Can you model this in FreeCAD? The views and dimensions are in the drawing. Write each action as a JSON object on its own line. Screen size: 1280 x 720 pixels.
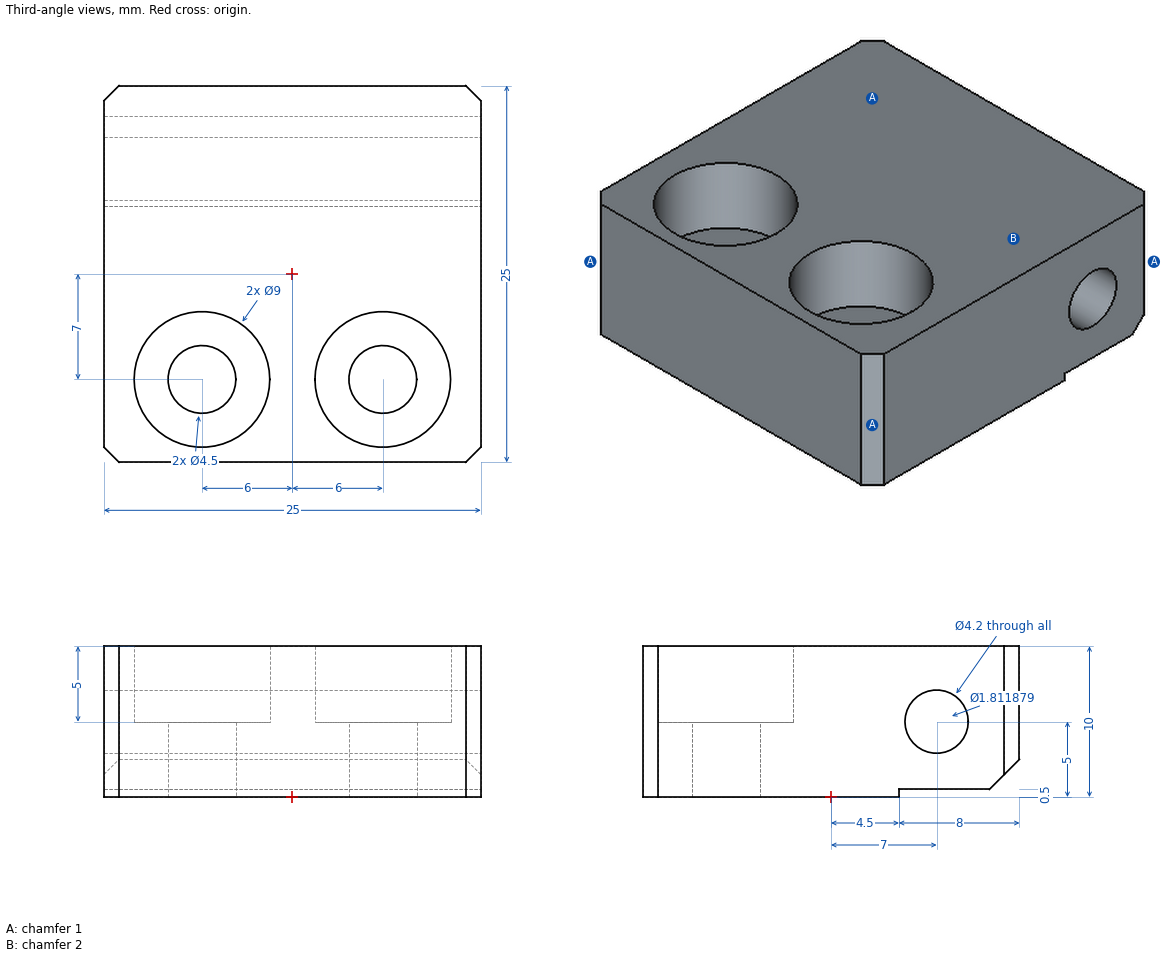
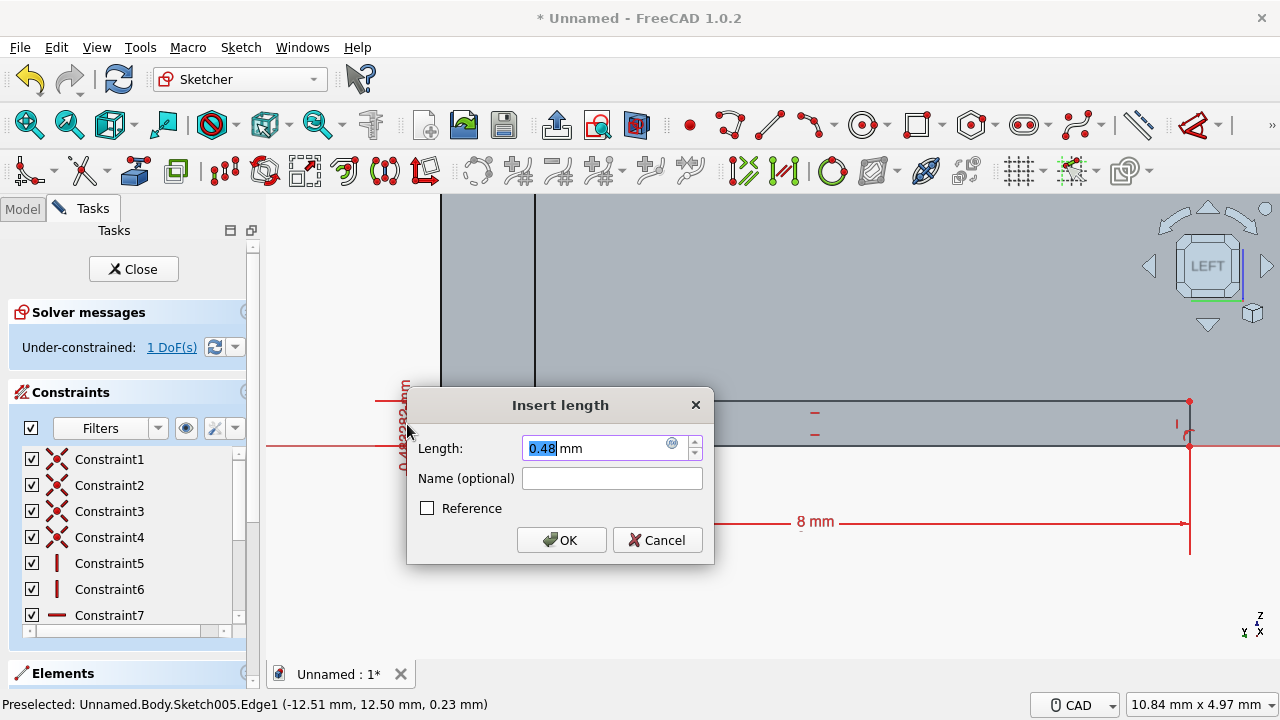
{"action": "type", "text": "0.5"}
{"action": "key", "text": "Return"}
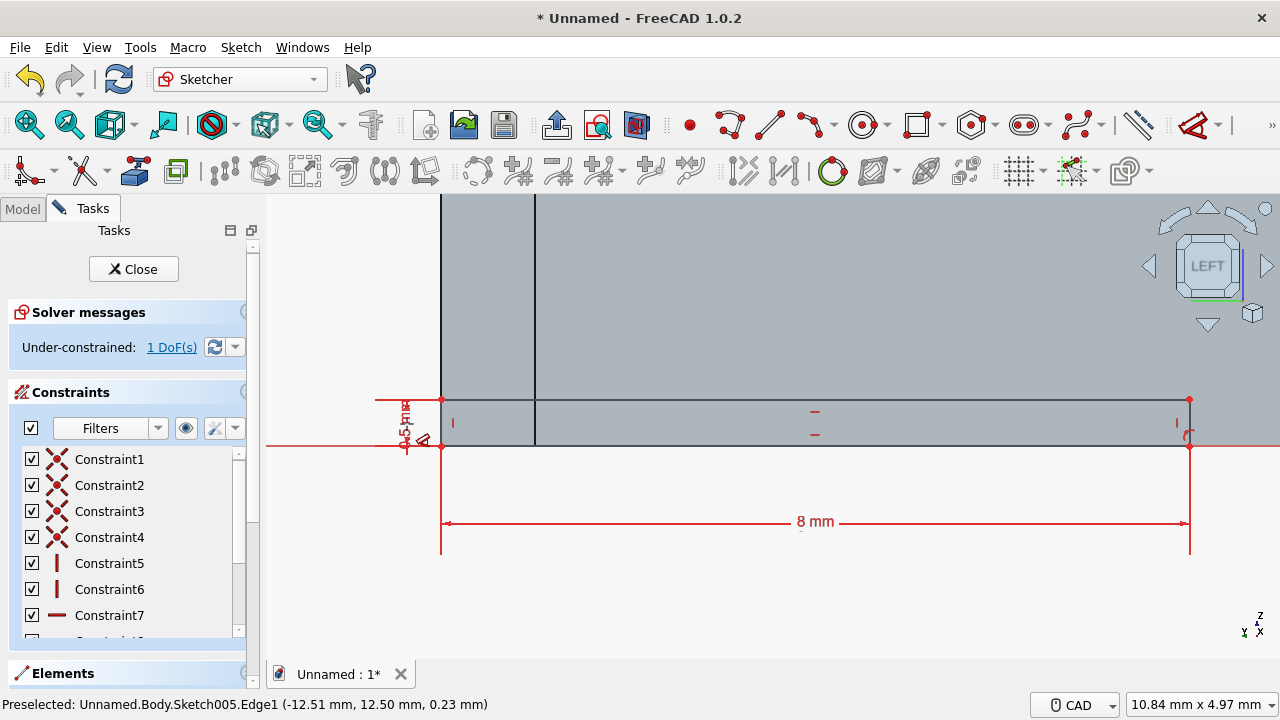
{"action": "scroll", "coordinate": [443, 429], "scroll_direction": "down", "scroll_amount": 4}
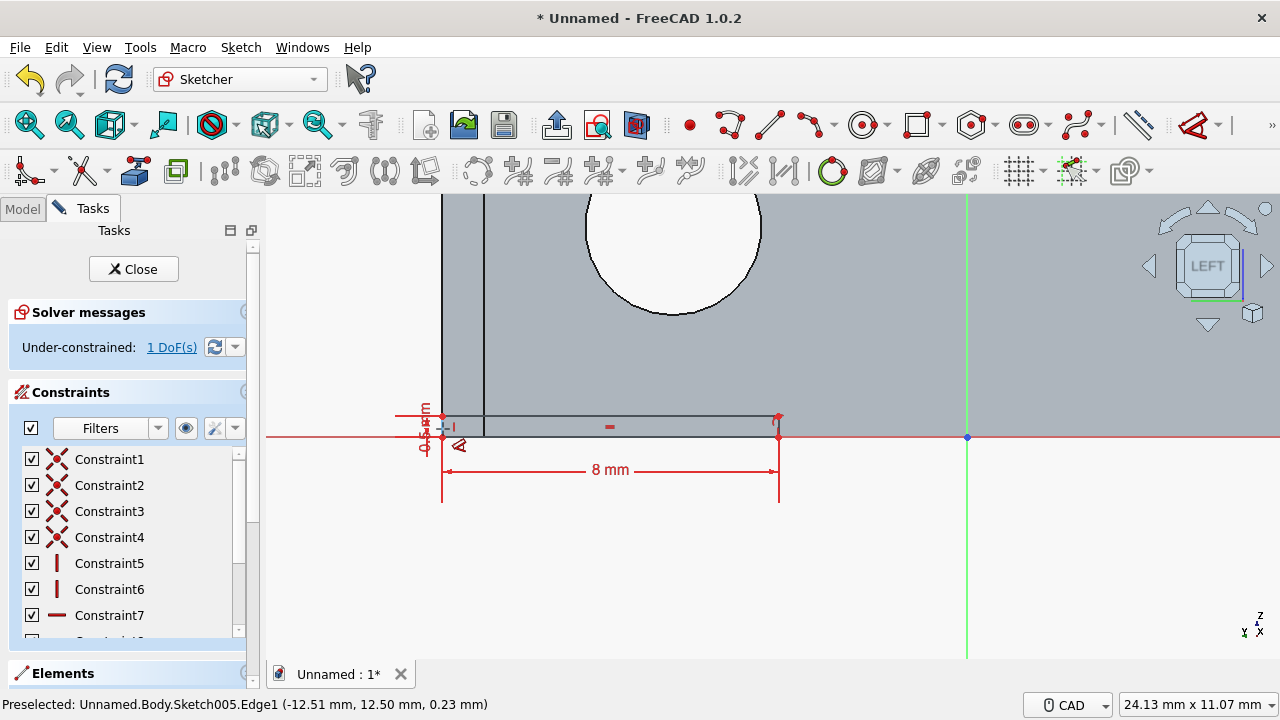
{"action": "left_click", "coordinate": [779, 437]}
{"action": "left_click", "coordinate": [873, 471]}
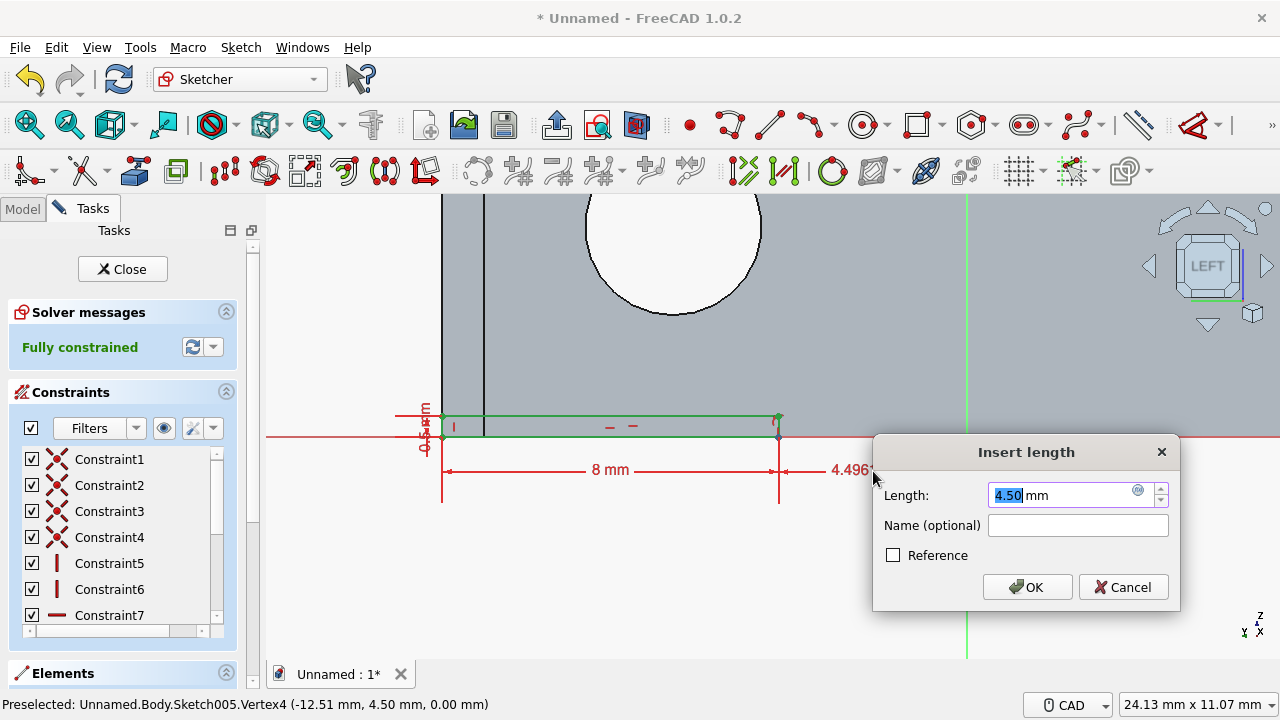
{"action": "type", "text": "4.5"}
{"action": "key", "text": "Return"}
{"action": "key", "text": "Escape"}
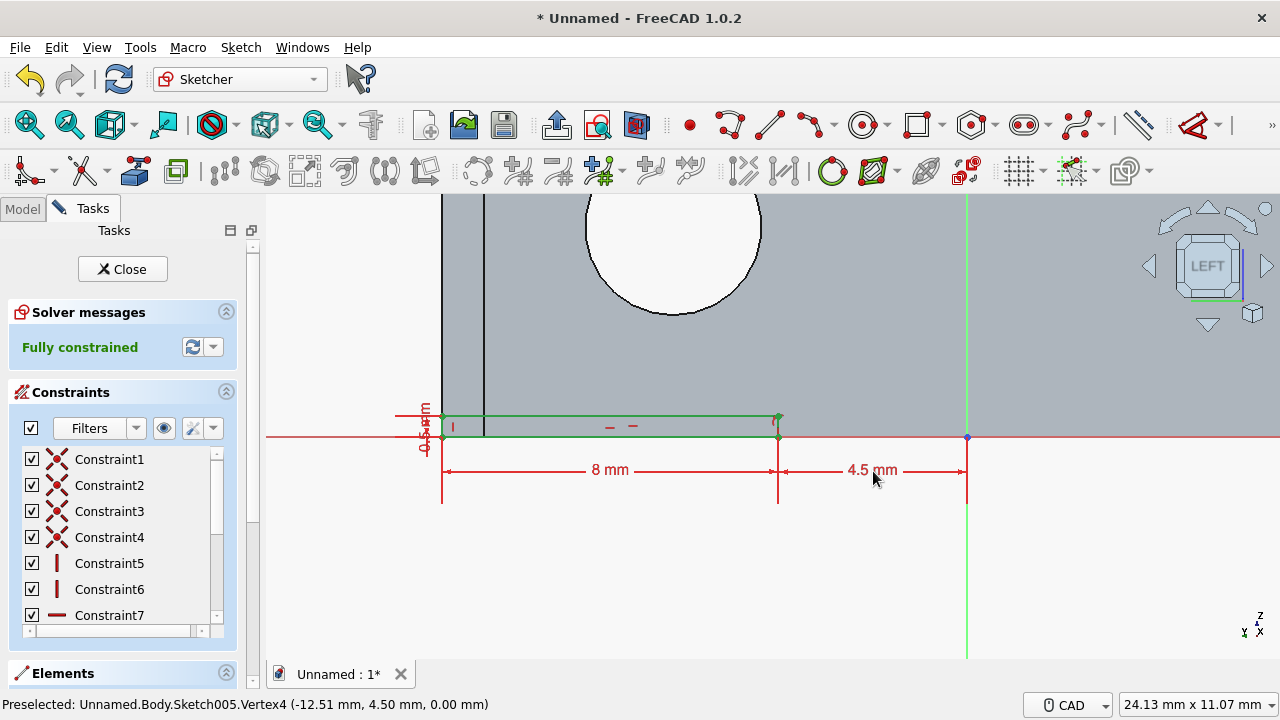
{"action": "left_click", "coordinate": [123, 269]}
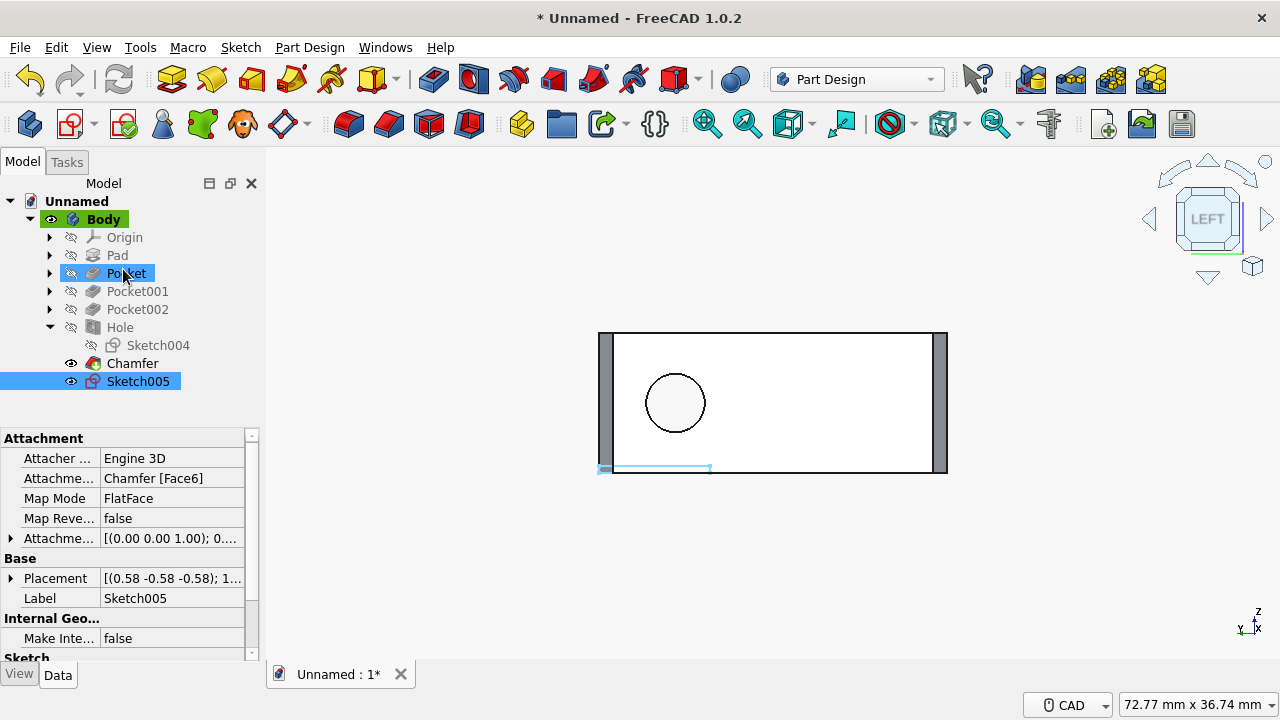
{"action": "left_click", "coordinate": [434, 80]}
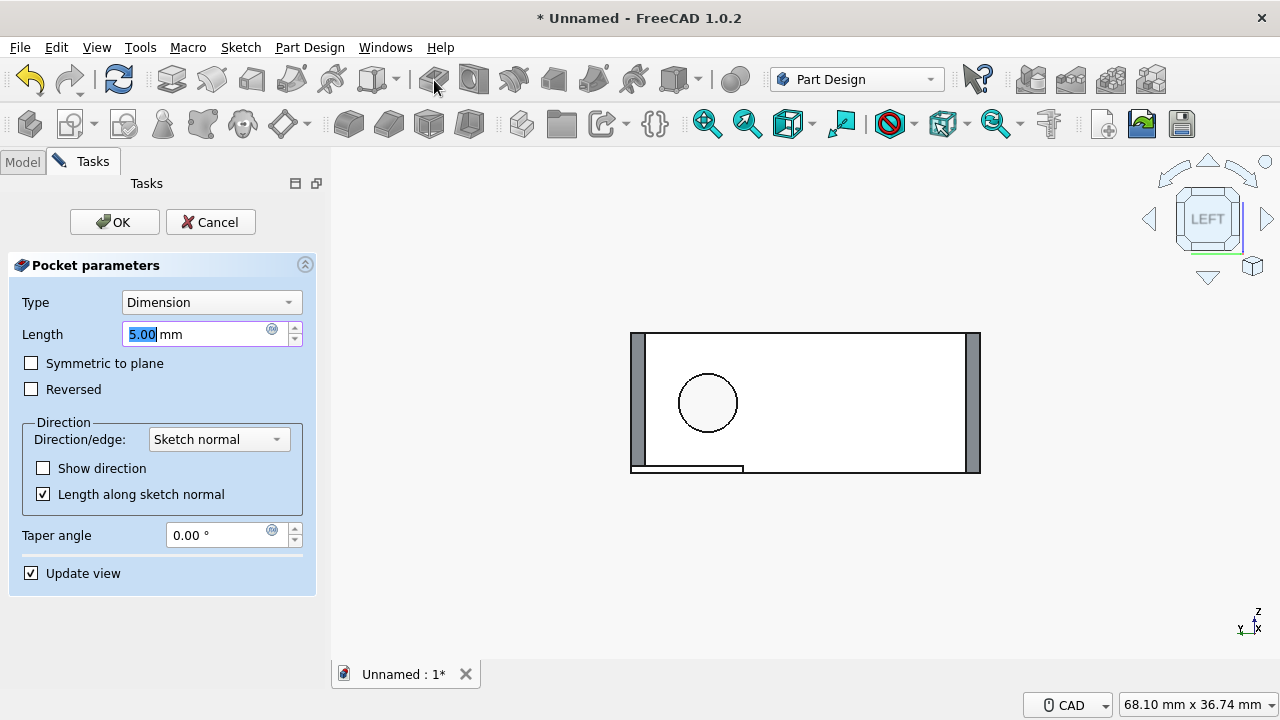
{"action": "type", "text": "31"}
{"action": "key", "text": "Tab"}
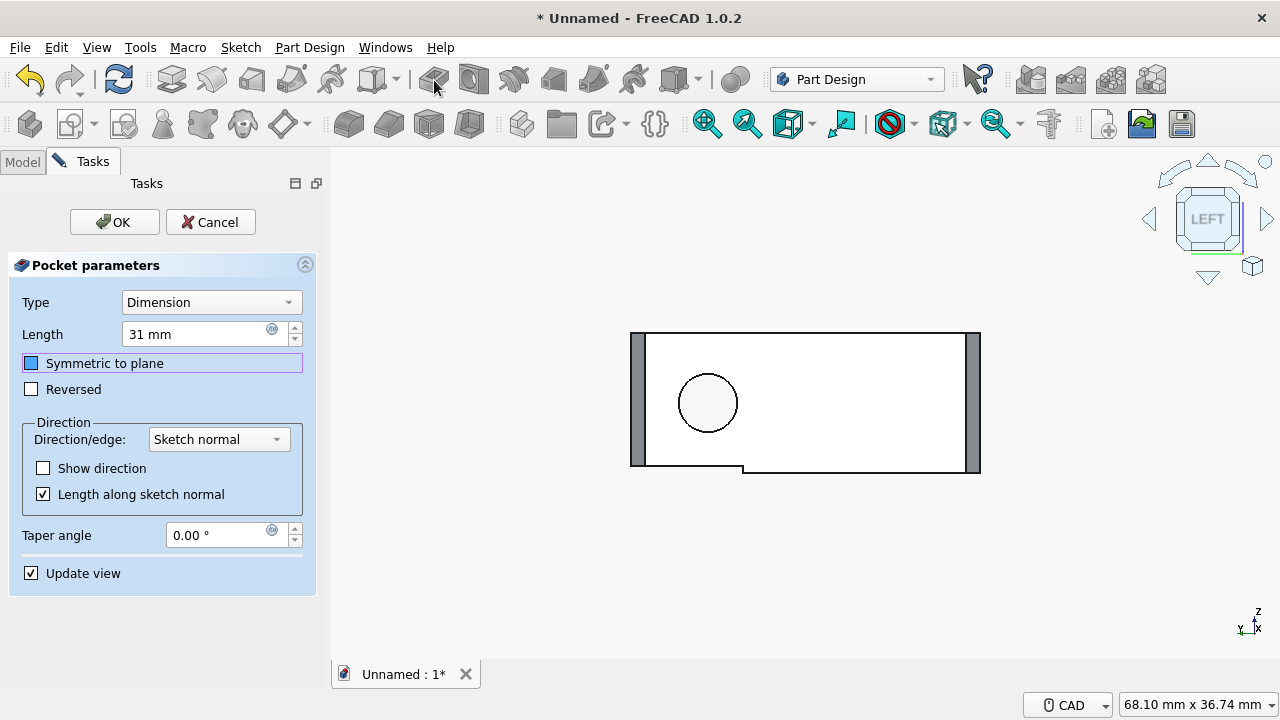
{"action": "left_click", "coordinate": [115, 222]}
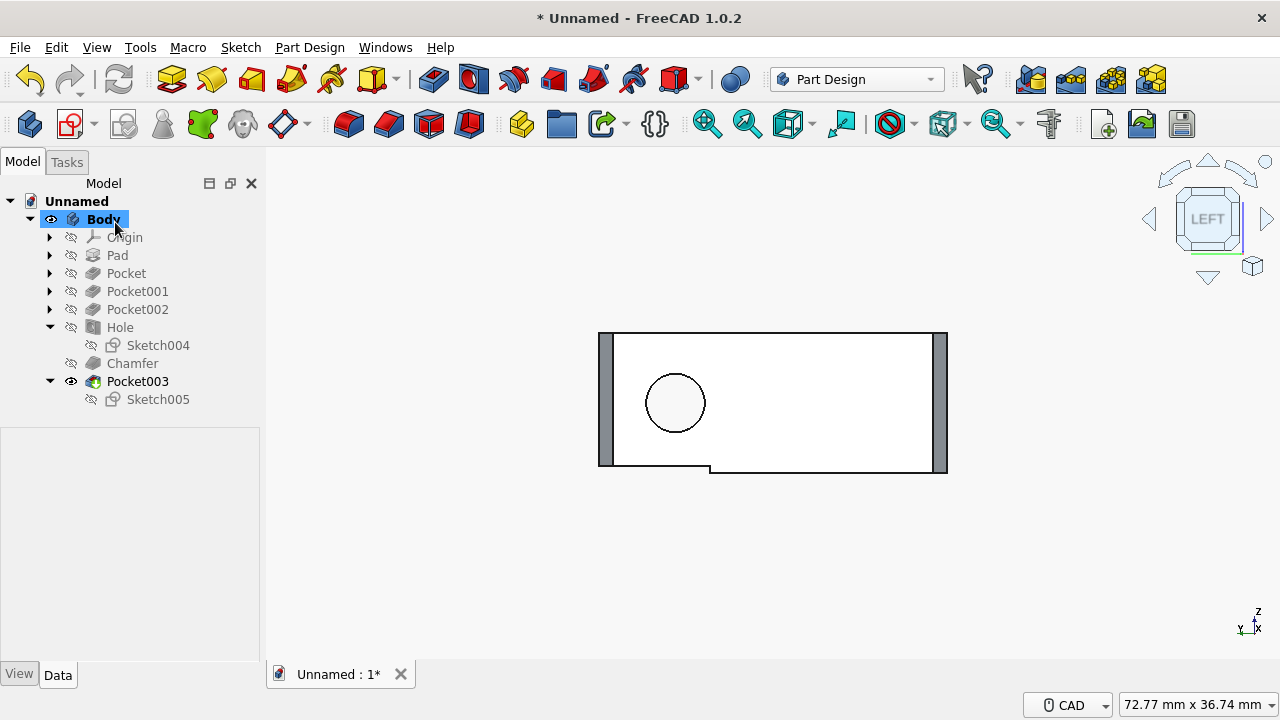
{"action": "left_click", "coordinate": [708, 124]}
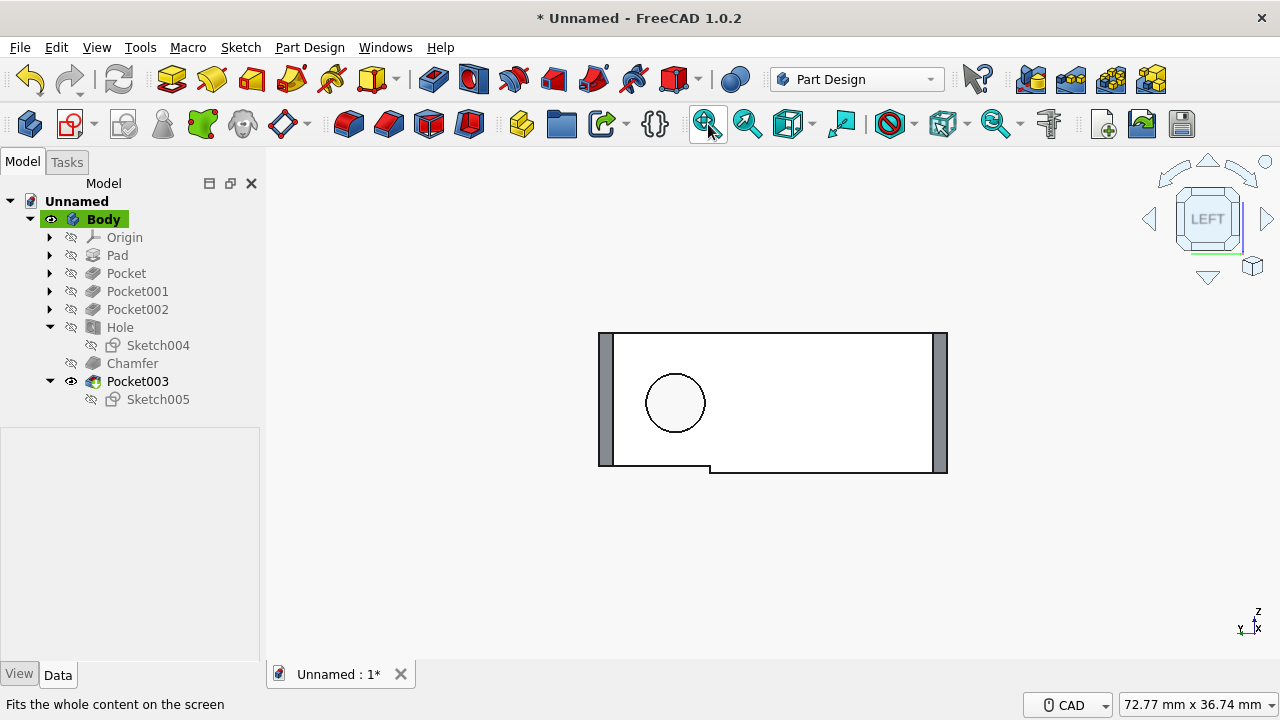
{"action": "key", "text": "0"}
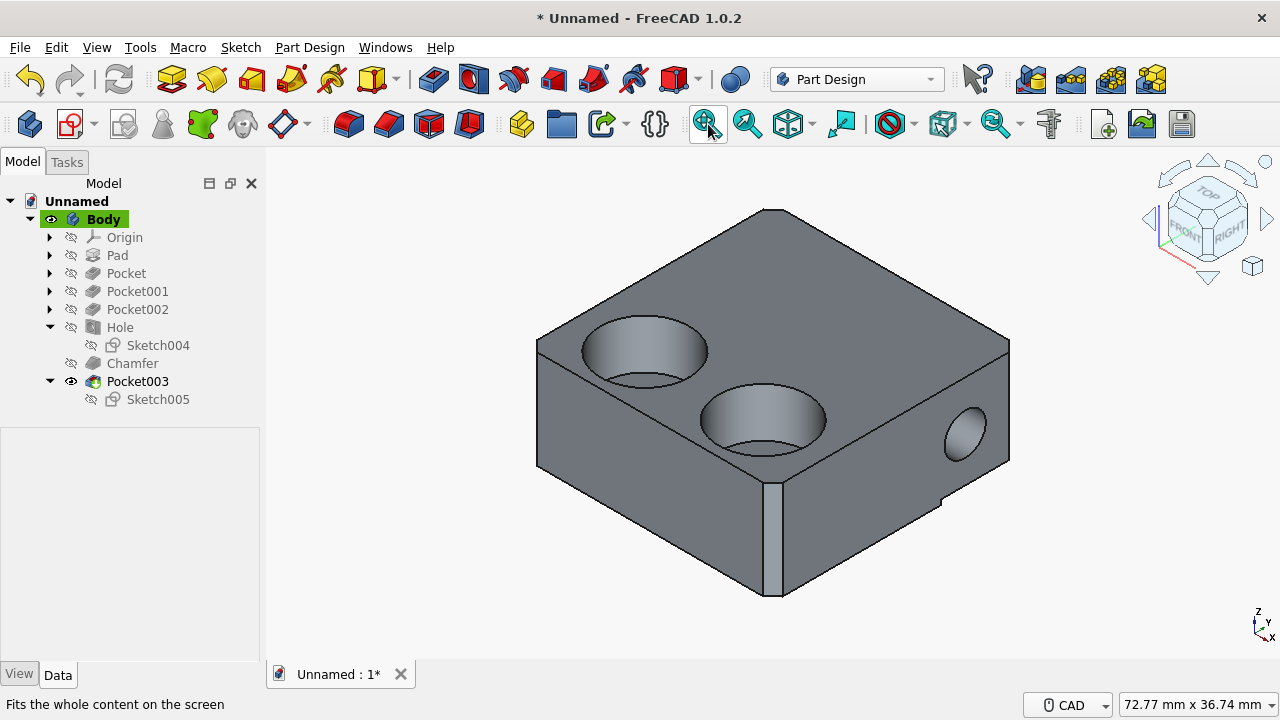
{"action": "key", "text": "2"}